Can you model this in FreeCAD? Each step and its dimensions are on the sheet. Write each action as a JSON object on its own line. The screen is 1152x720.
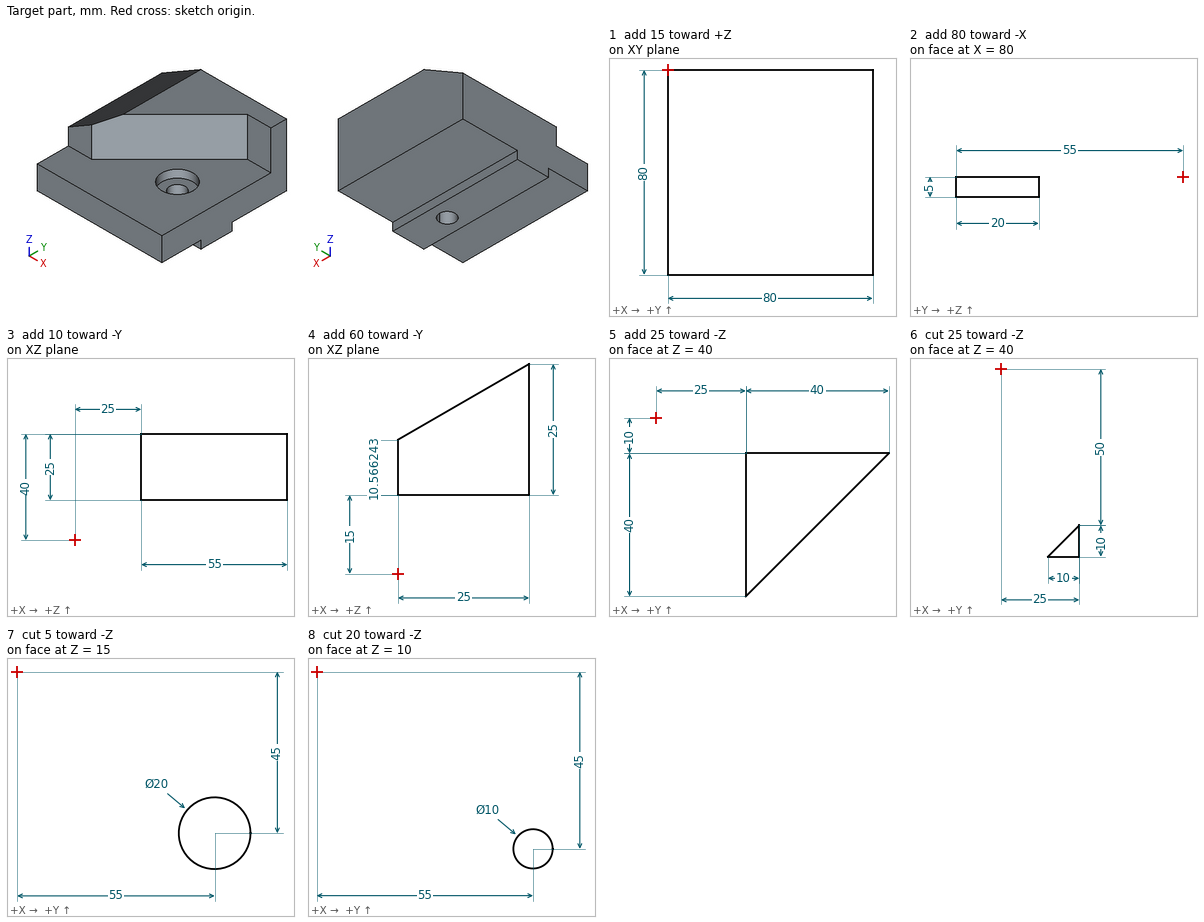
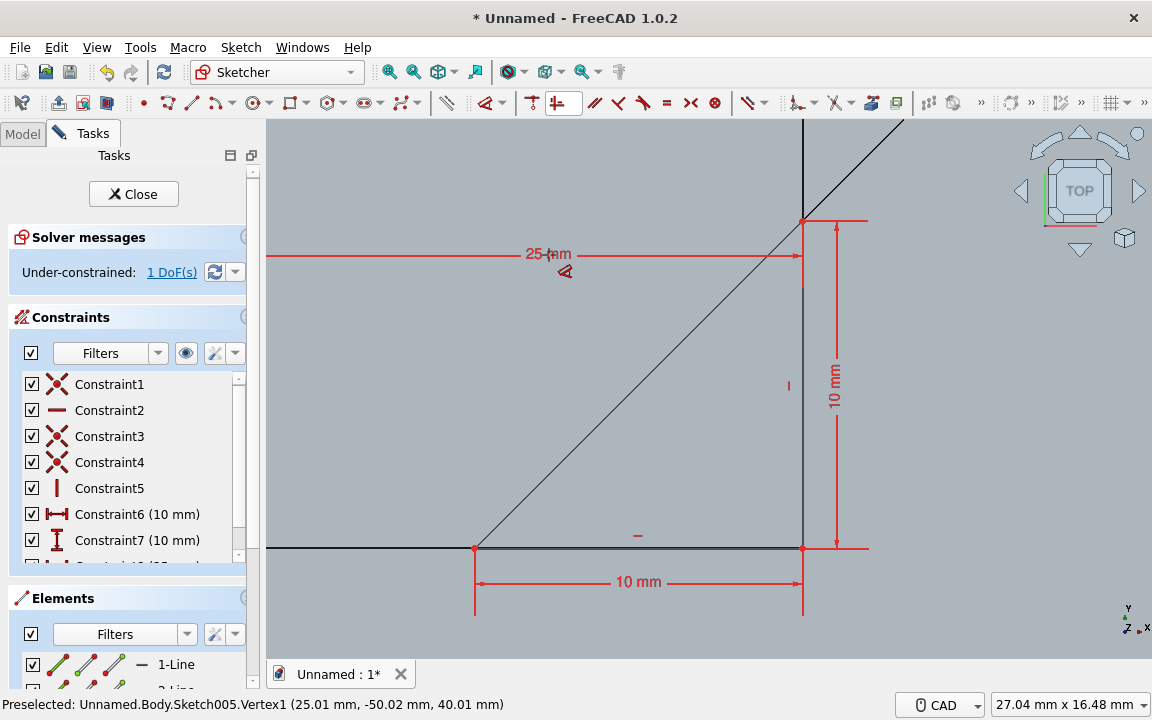
{"action": "left_click", "coordinate": [803, 221]}
{"action": "left_click", "coordinate": [837, 184]}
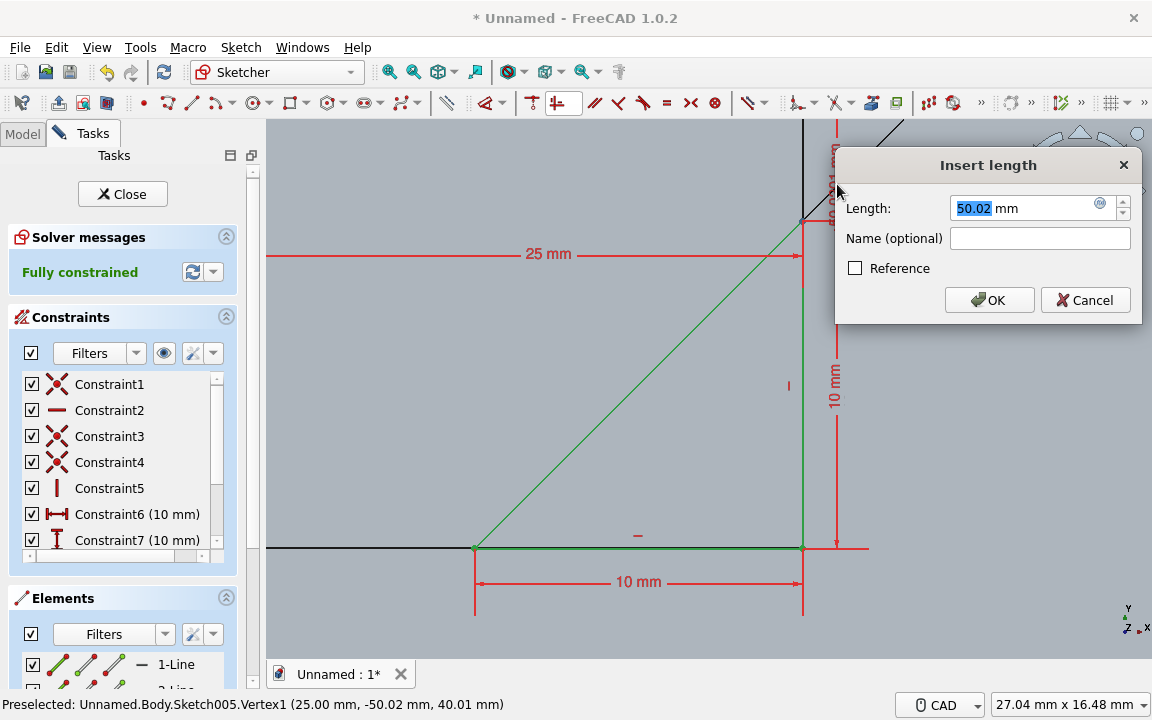
{"action": "type", "text": "50"}
{"action": "key", "text": "Return"}
{"action": "key", "text": "Escape"}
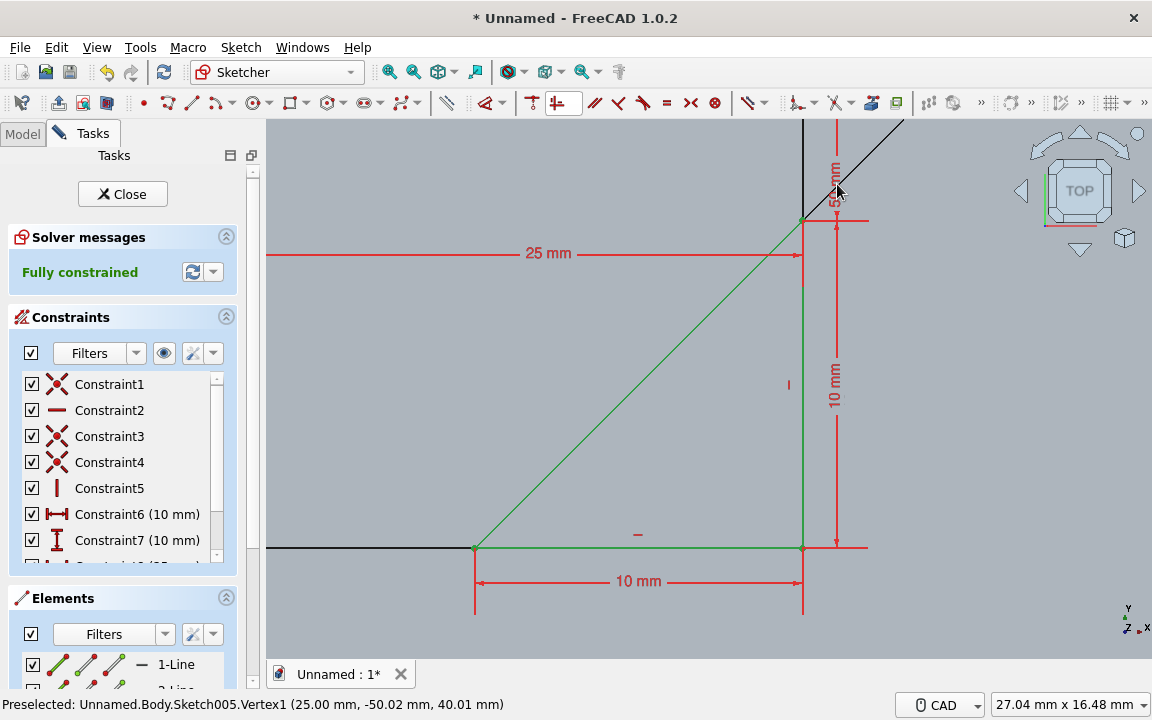
{"action": "left_click", "coordinate": [123, 194]}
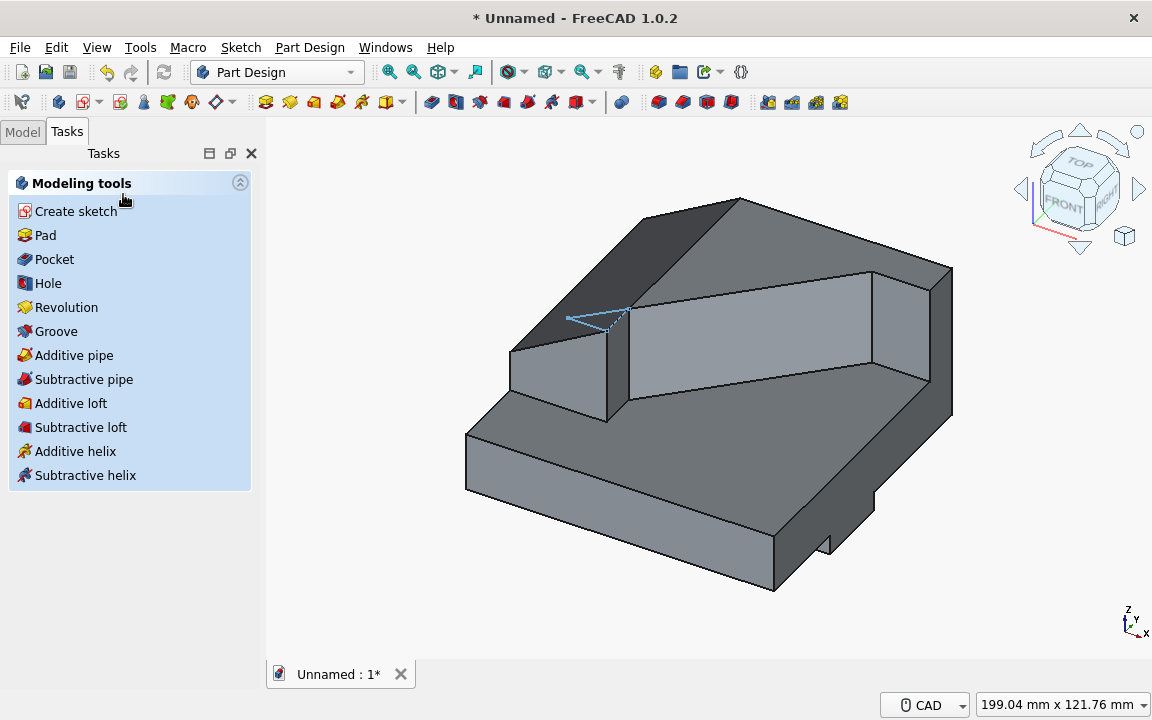
{"action": "left_click", "coordinate": [432, 102]}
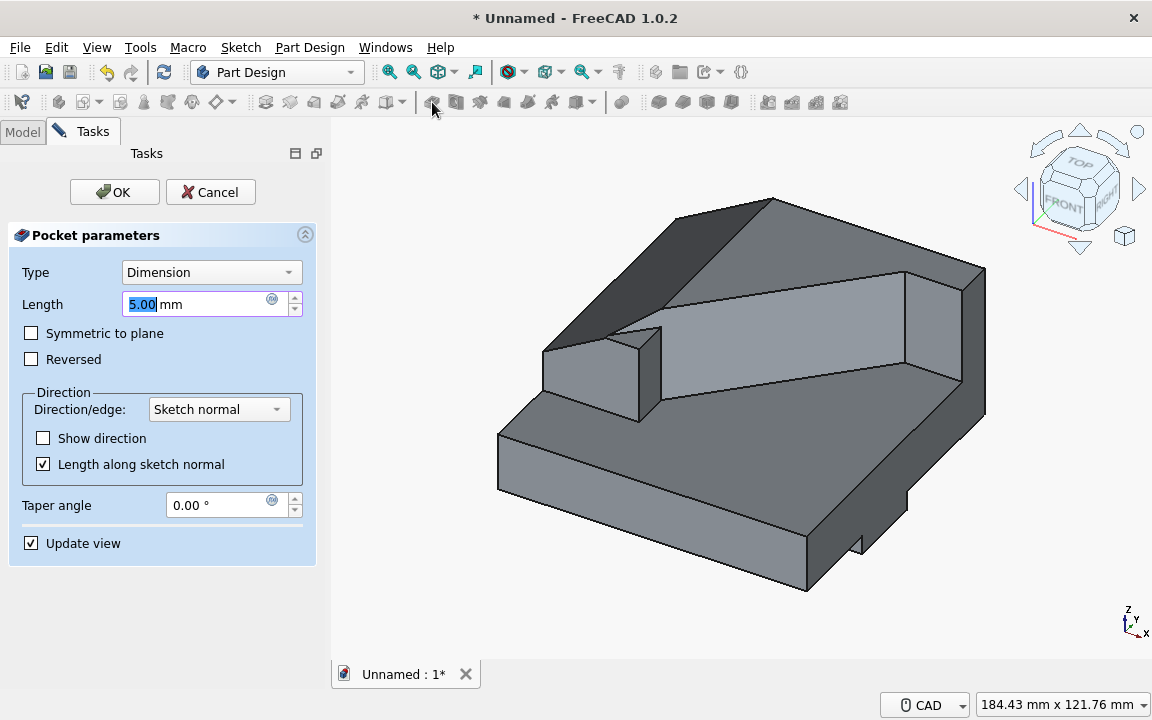
{"action": "type", "text": "25"}
{"action": "key", "text": "Tab"}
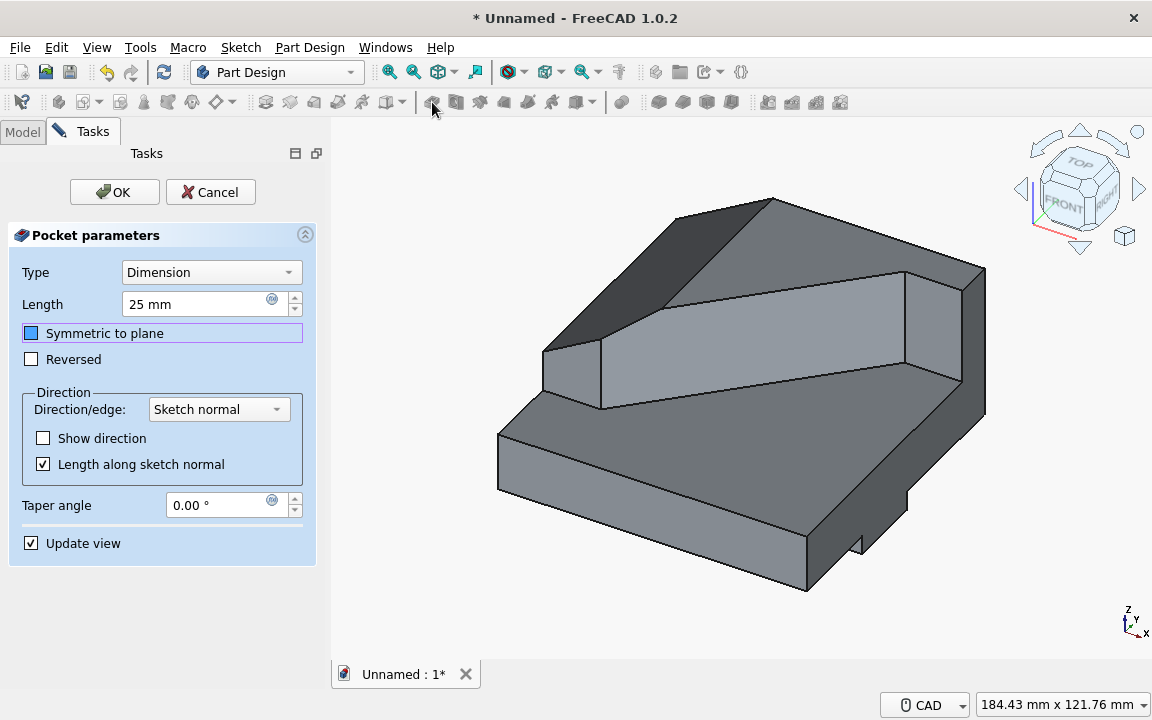
{"action": "left_click", "coordinate": [115, 192]}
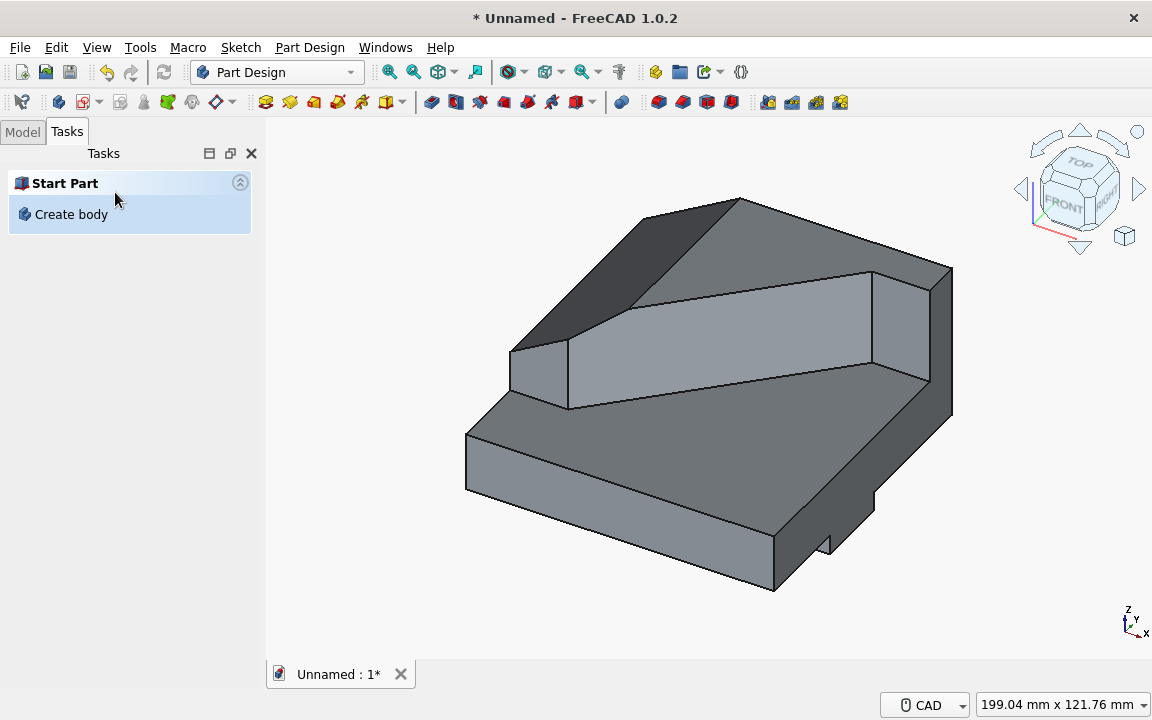
{"action": "left_click", "coordinate": [720, 444]}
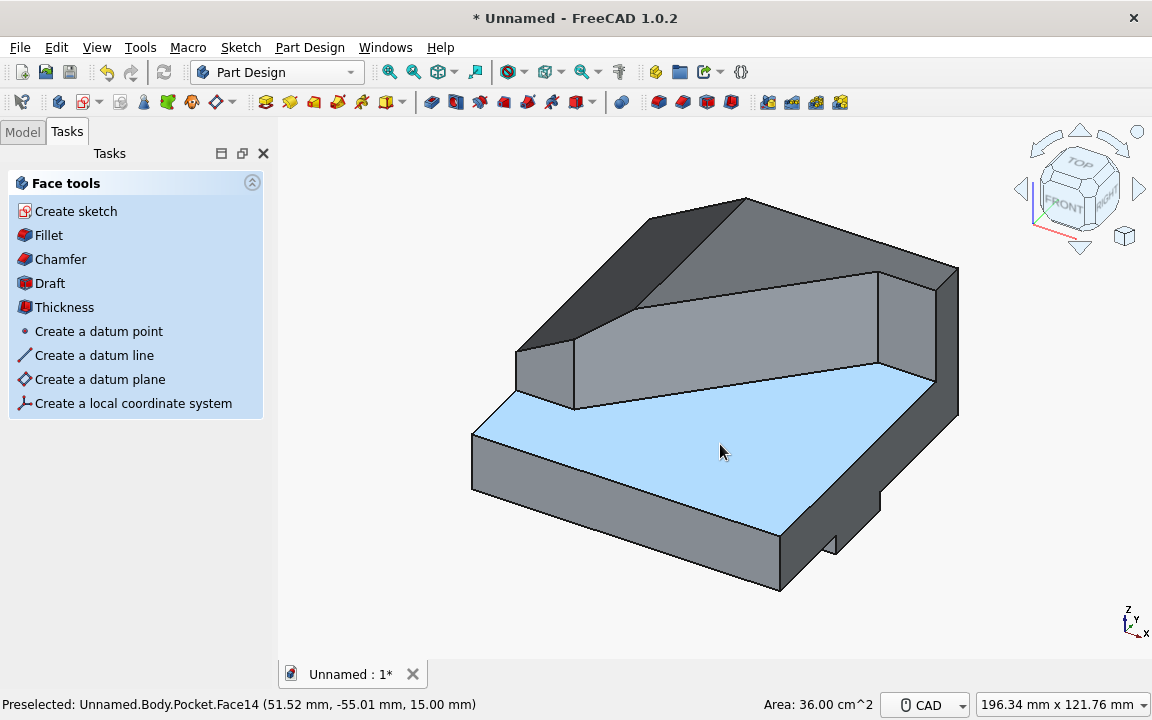
{"action": "left_click", "coordinate": [84, 102]}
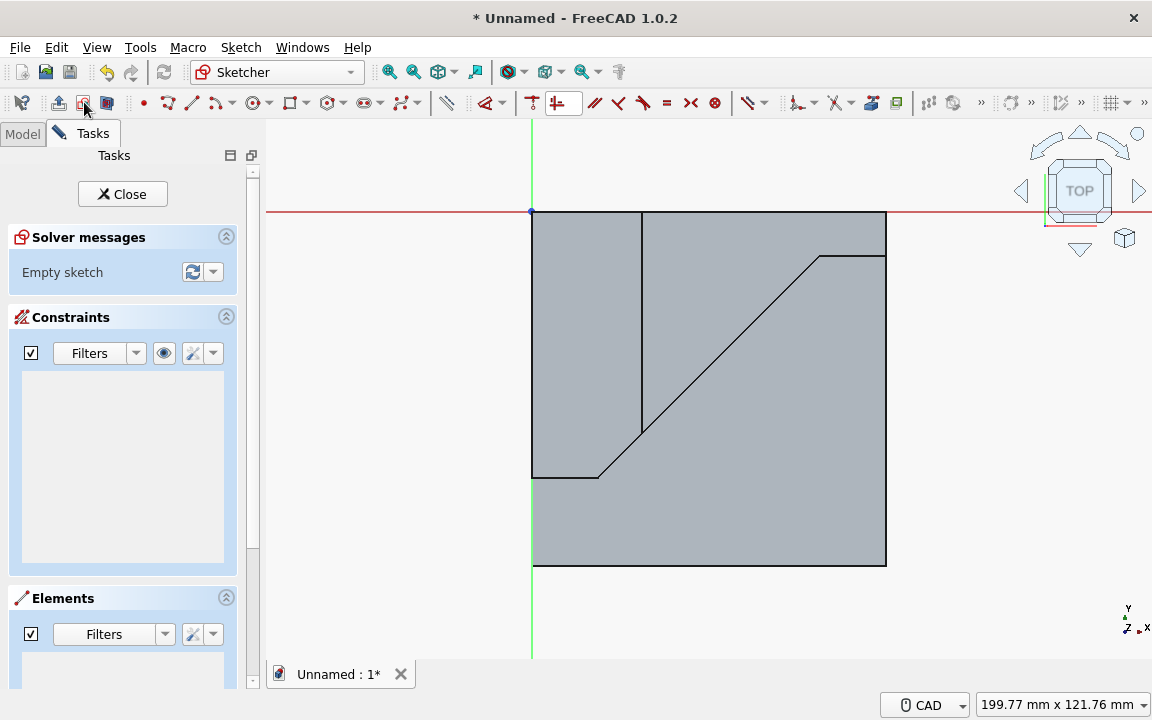
{"action": "scroll", "coordinate": [820, 418], "scroll_direction": "up", "scroll_amount": 7}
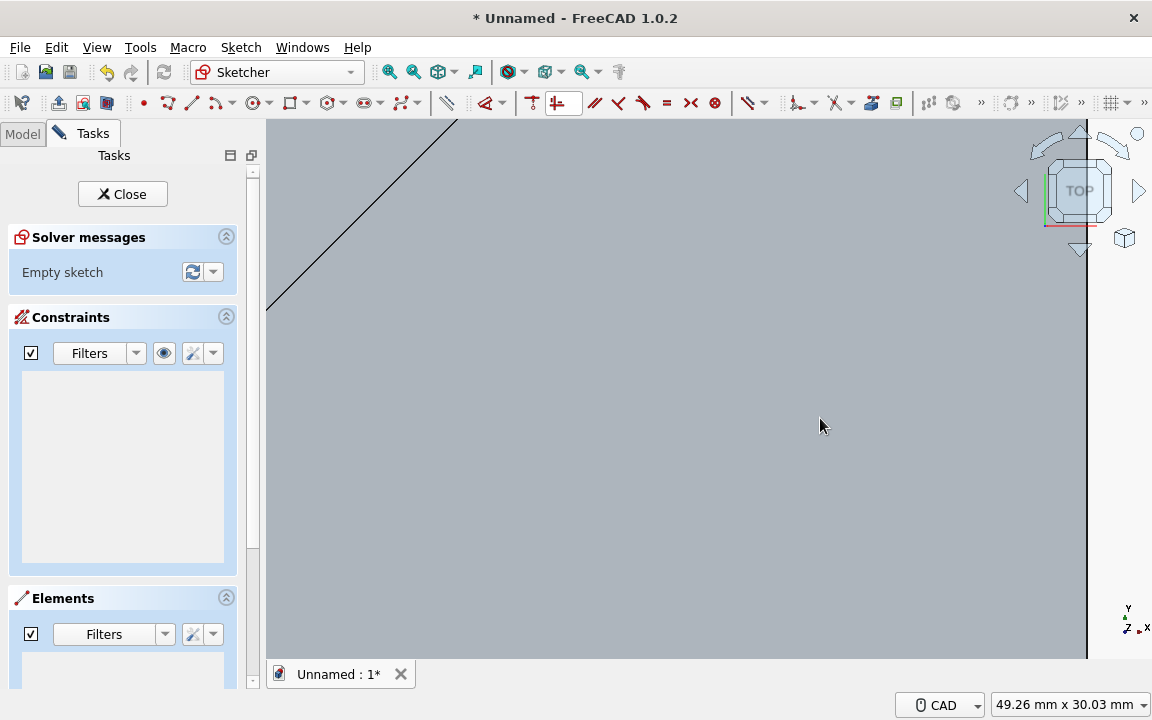
{"action": "left_click", "coordinate": [254, 104]}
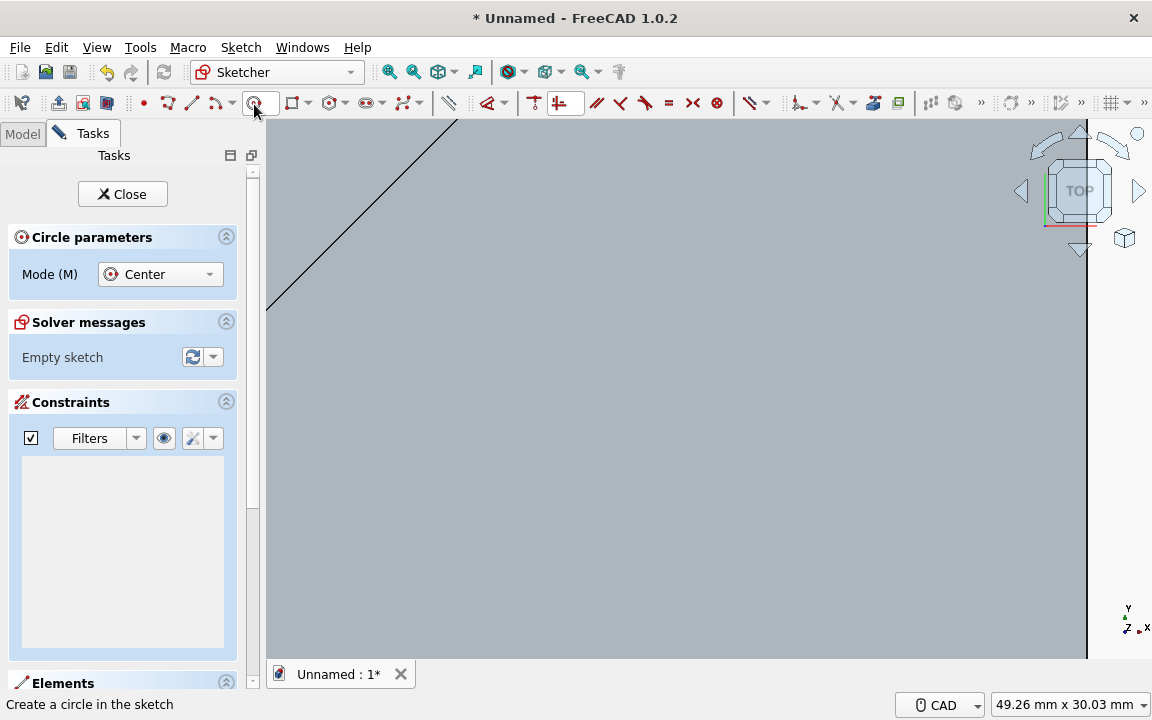
{"action": "left_click", "coordinate": [638, 389]}
{"action": "left_click", "coordinate": [765, 261]}
{"action": "key", "text": "Escape"}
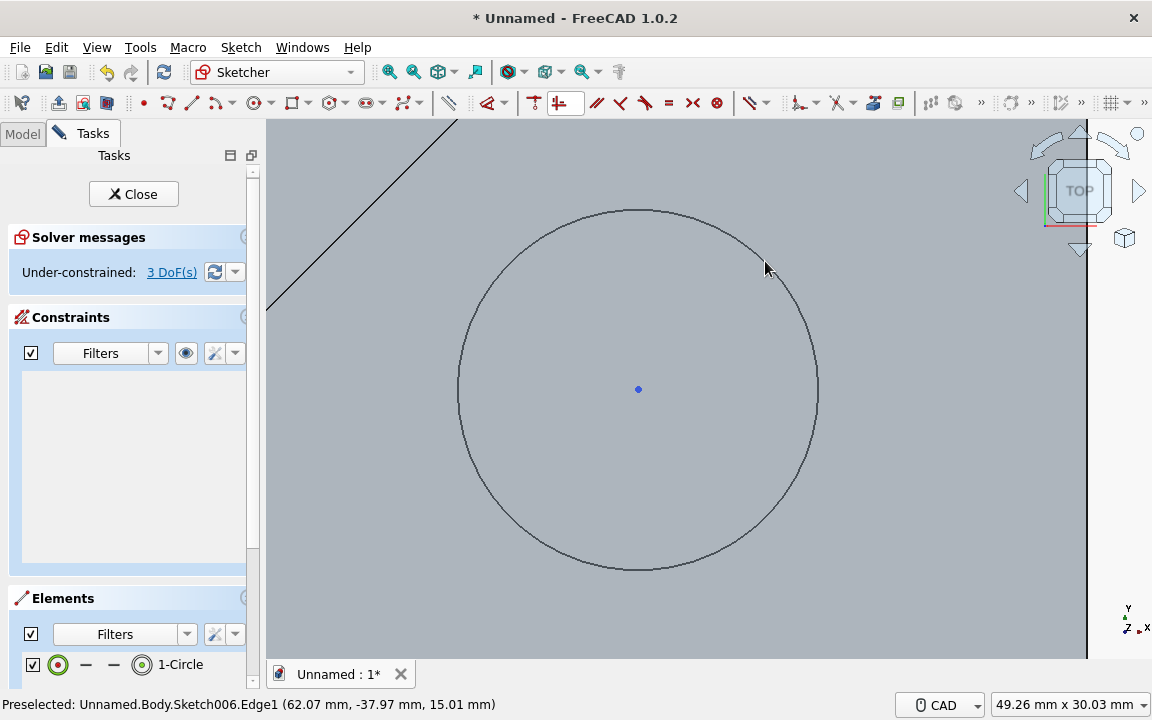
{"action": "left_click", "coordinate": [488, 104]}